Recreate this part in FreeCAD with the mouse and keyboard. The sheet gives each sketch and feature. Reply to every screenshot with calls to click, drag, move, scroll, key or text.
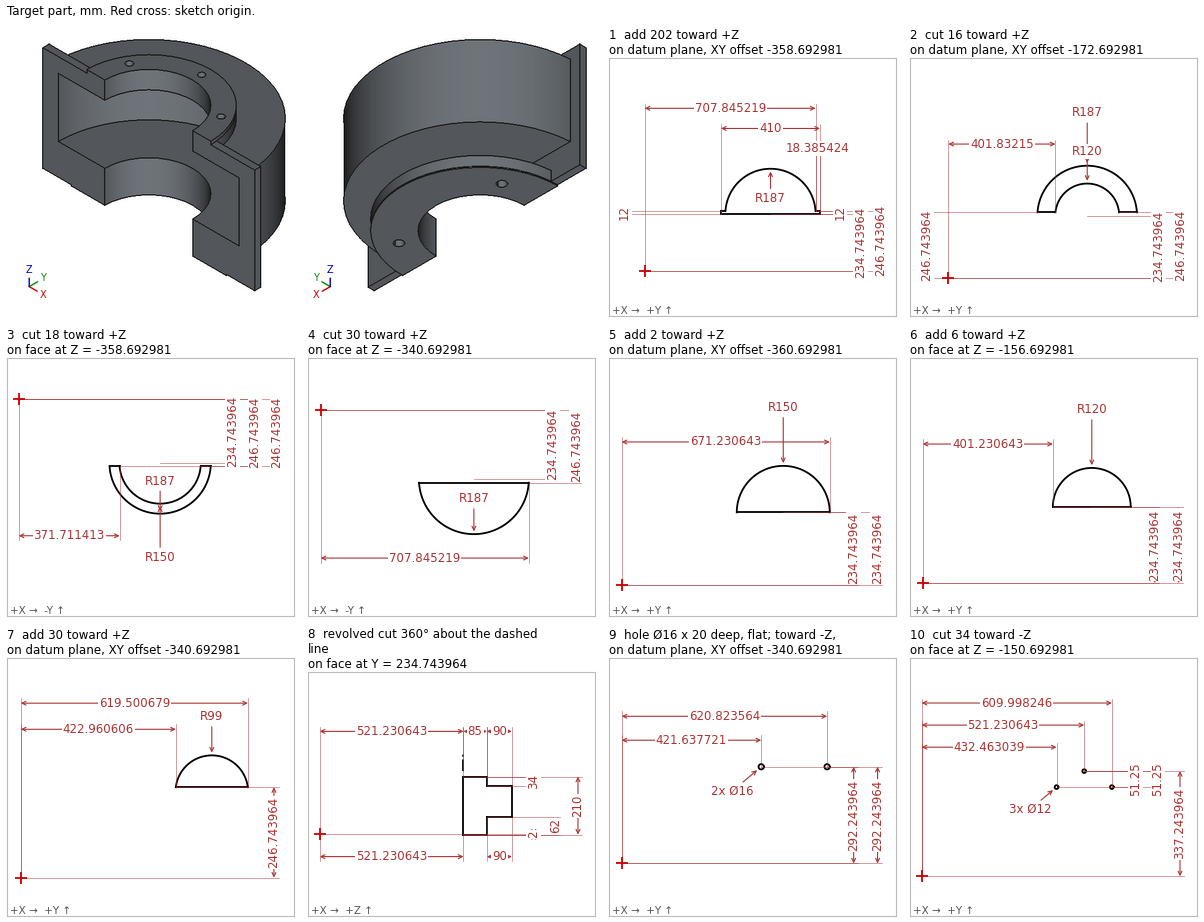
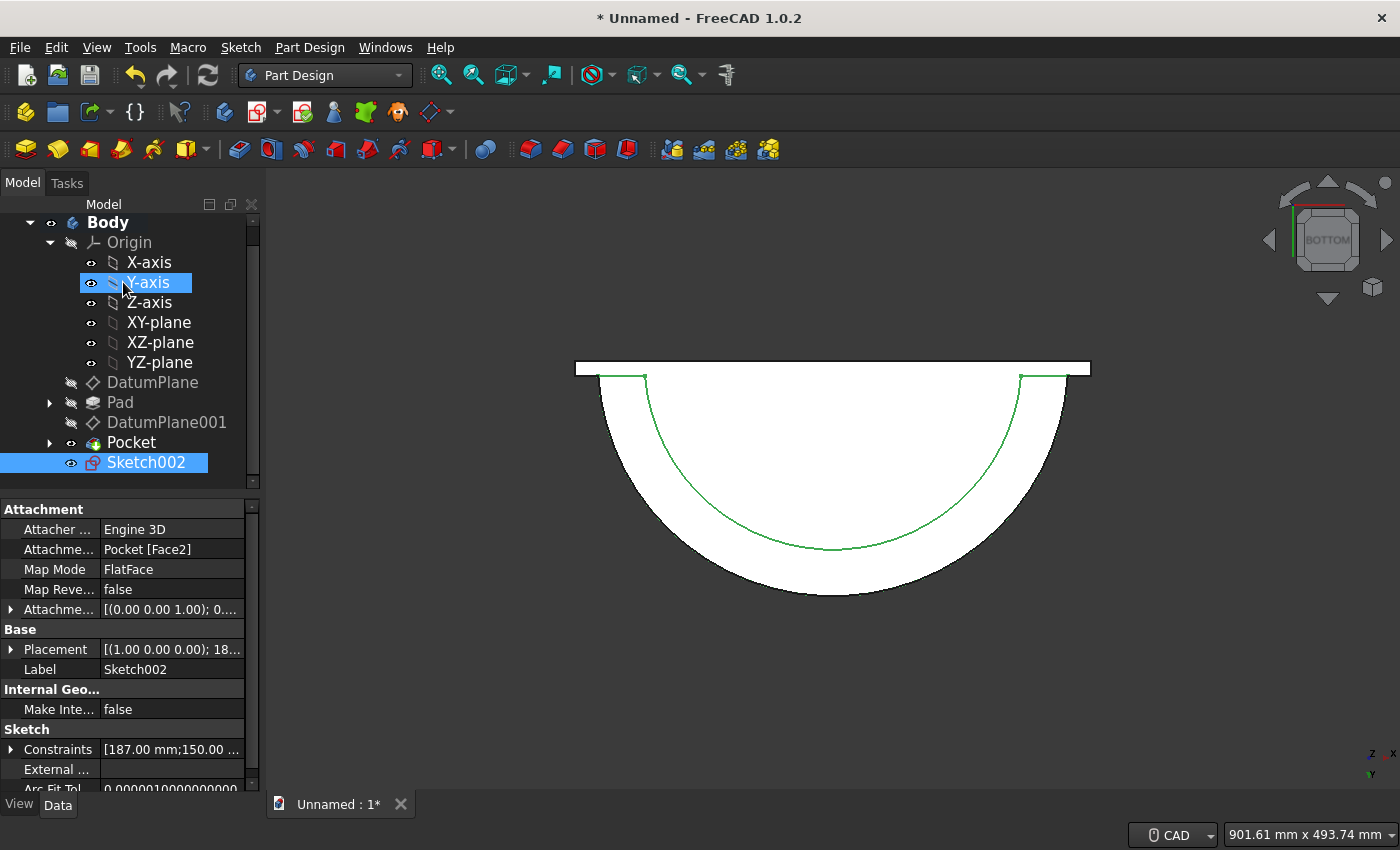
click(240, 150)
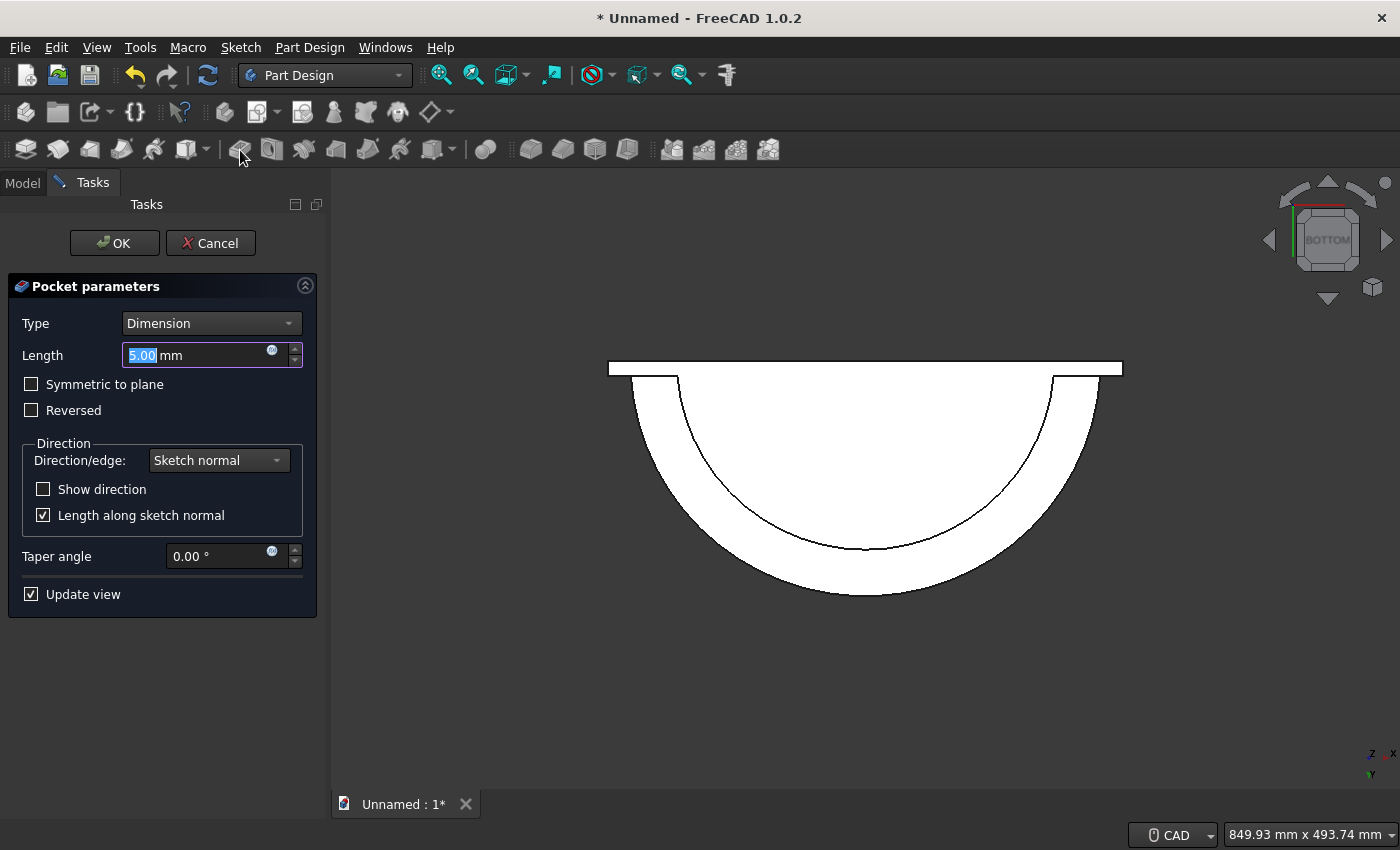
text(18)
key(Tab)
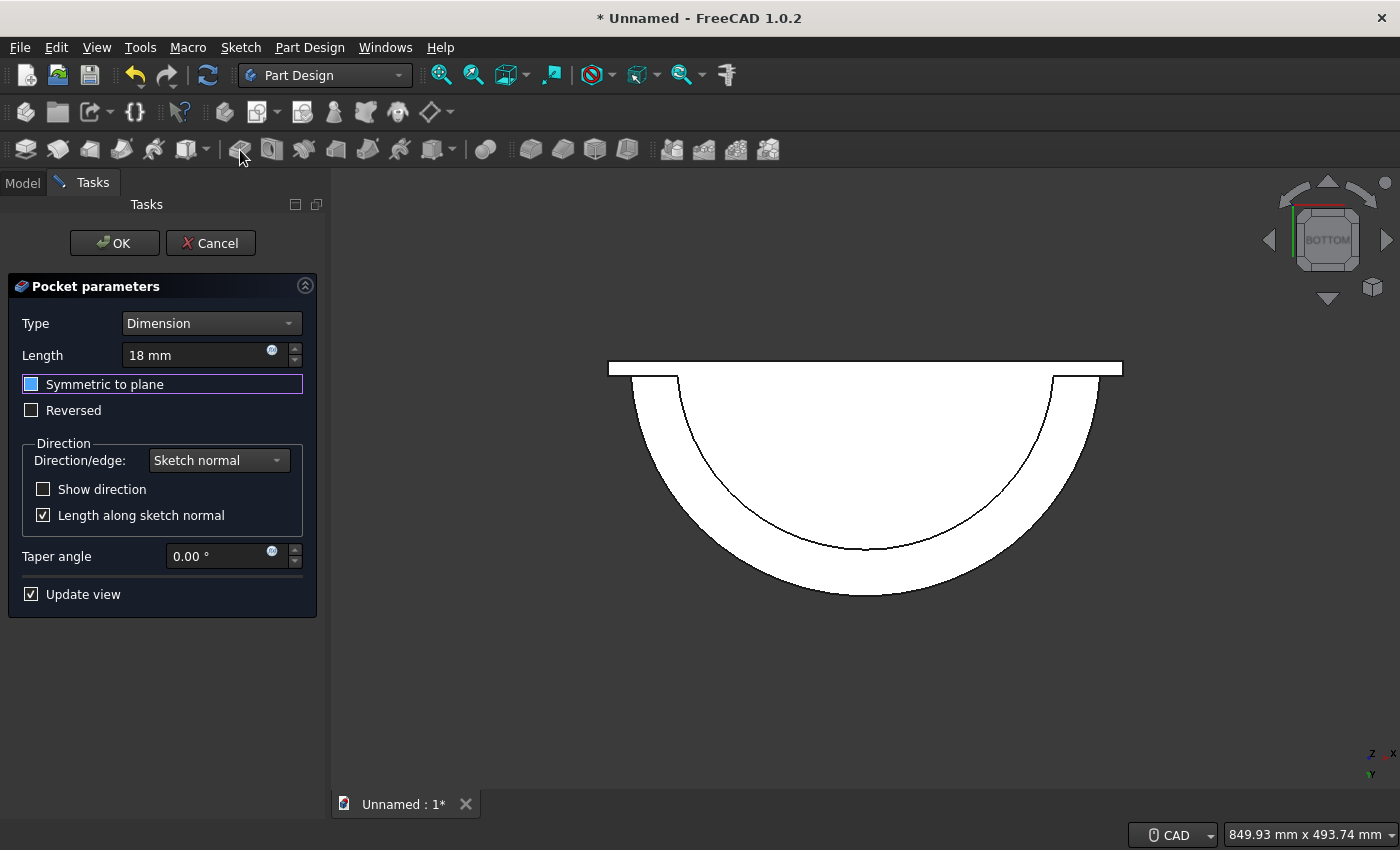
click(115, 243)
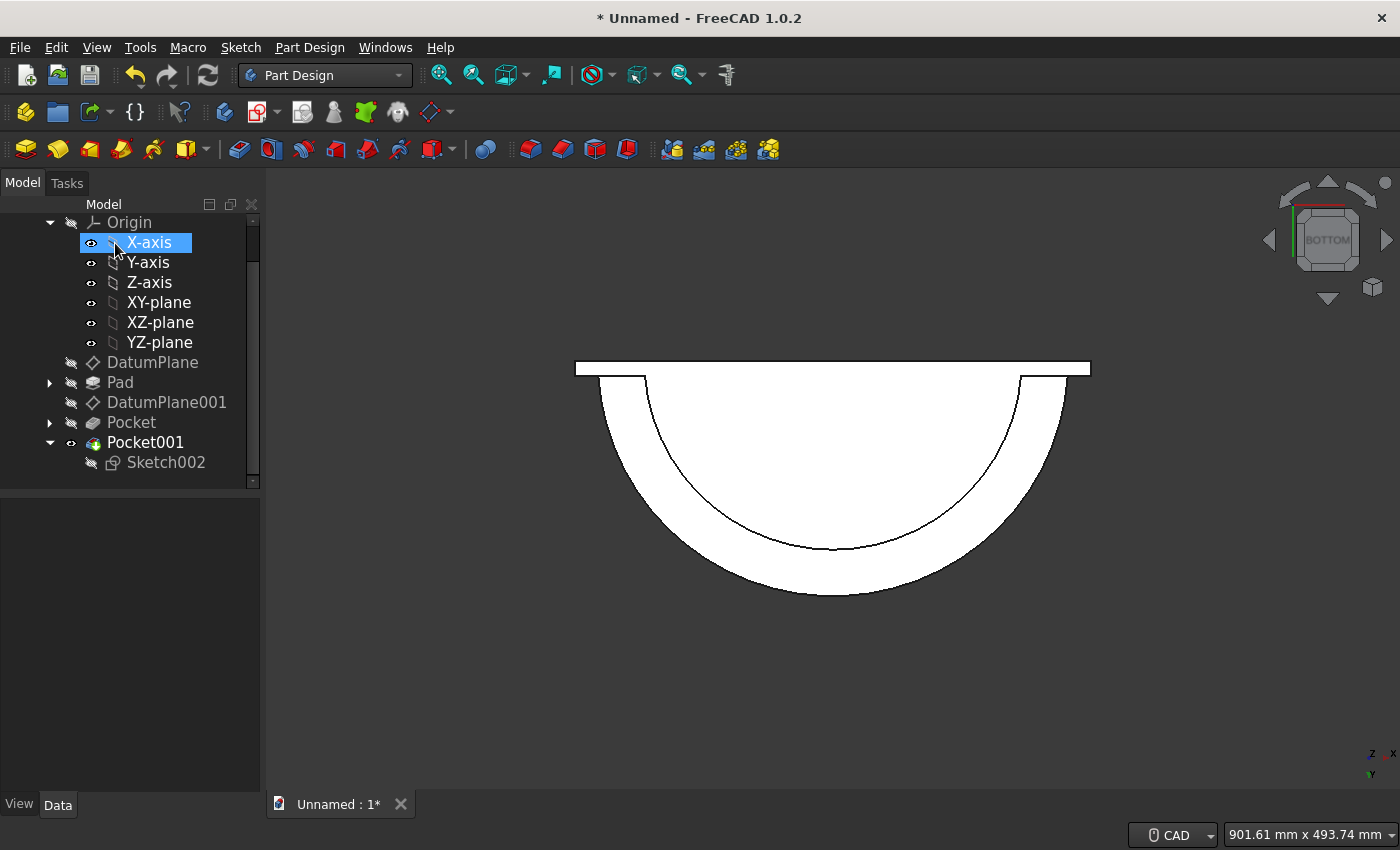
click(632, 422)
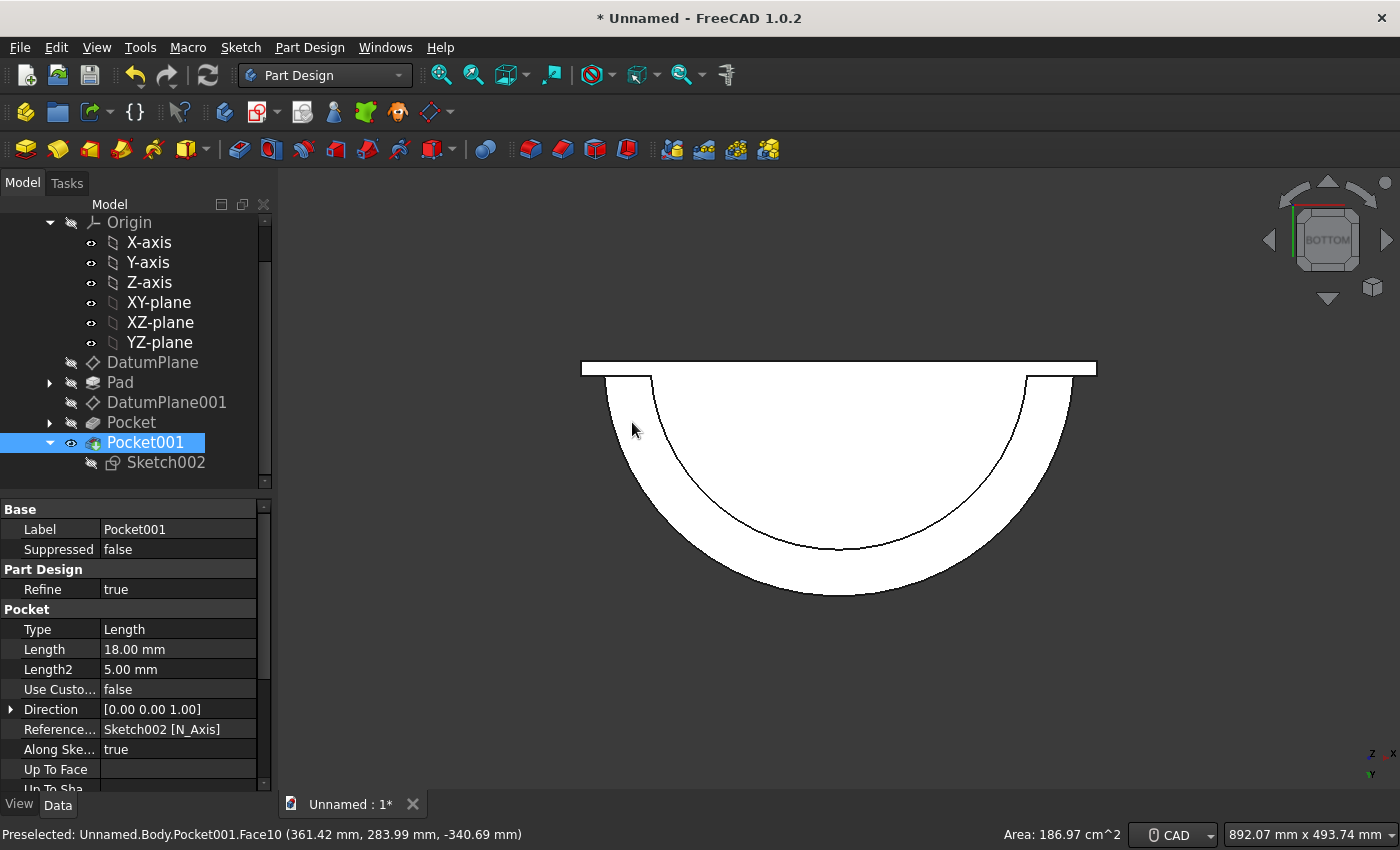
click(258, 112)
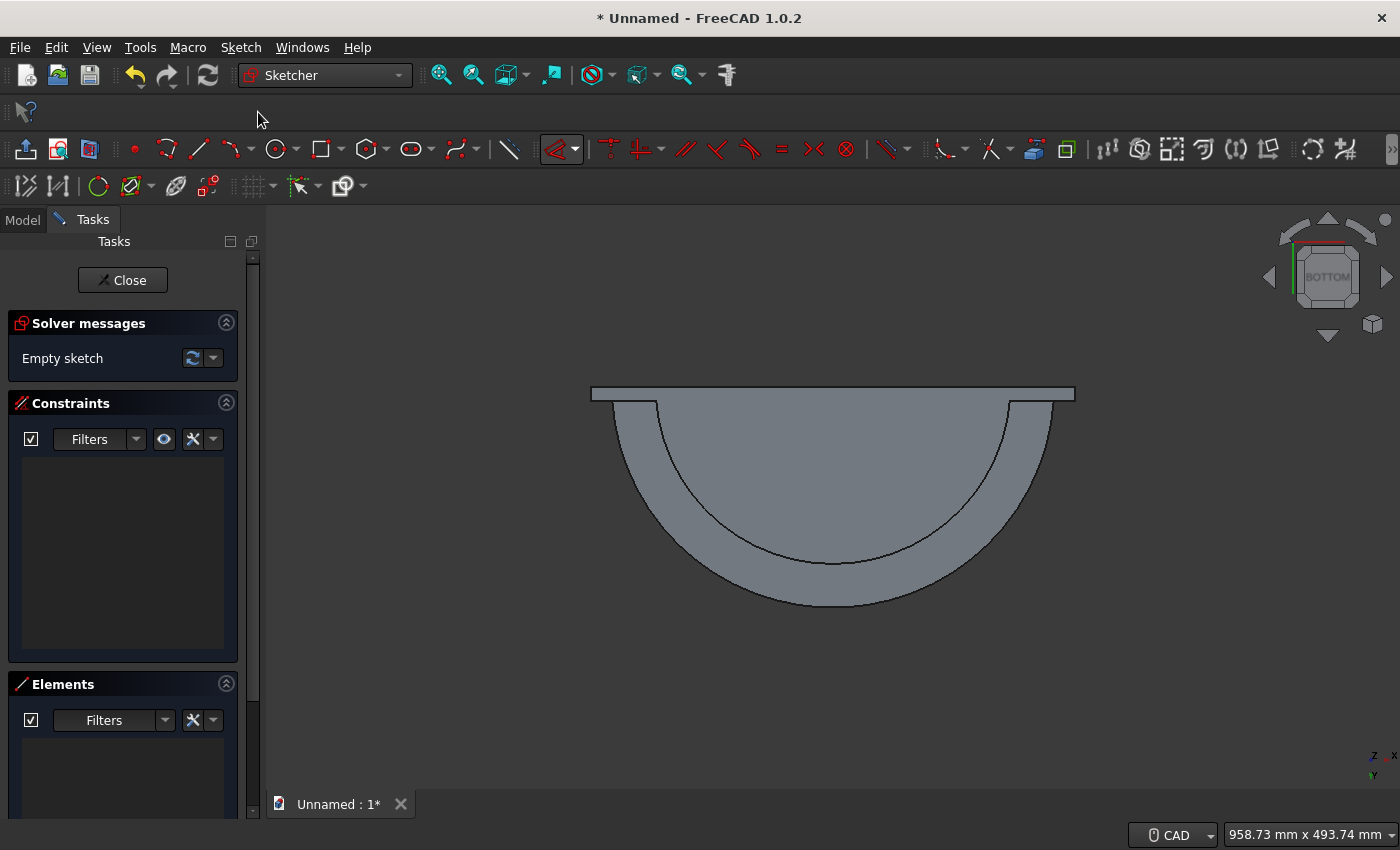
scroll(1028, 761, down, 2)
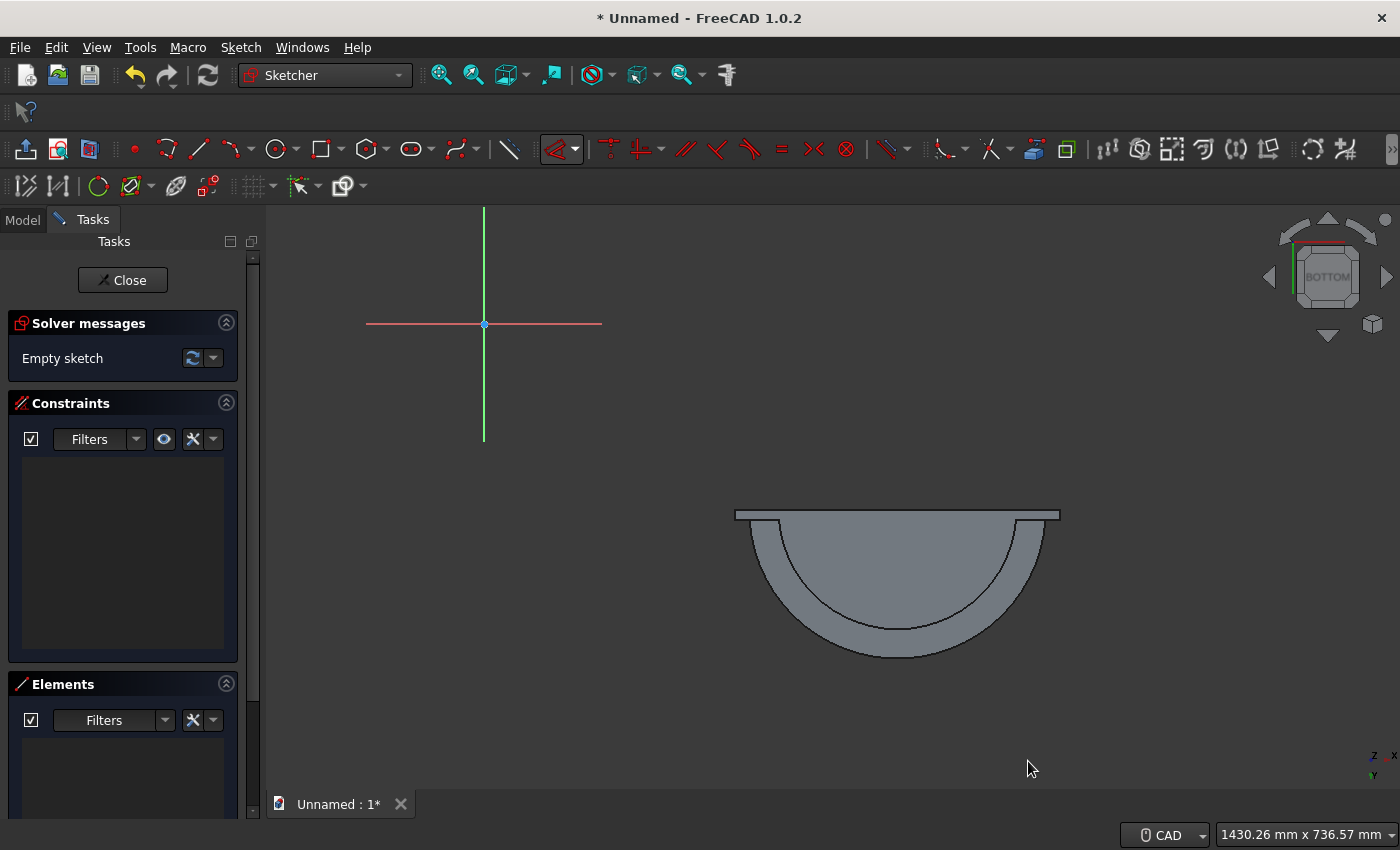
key(g)
key(l)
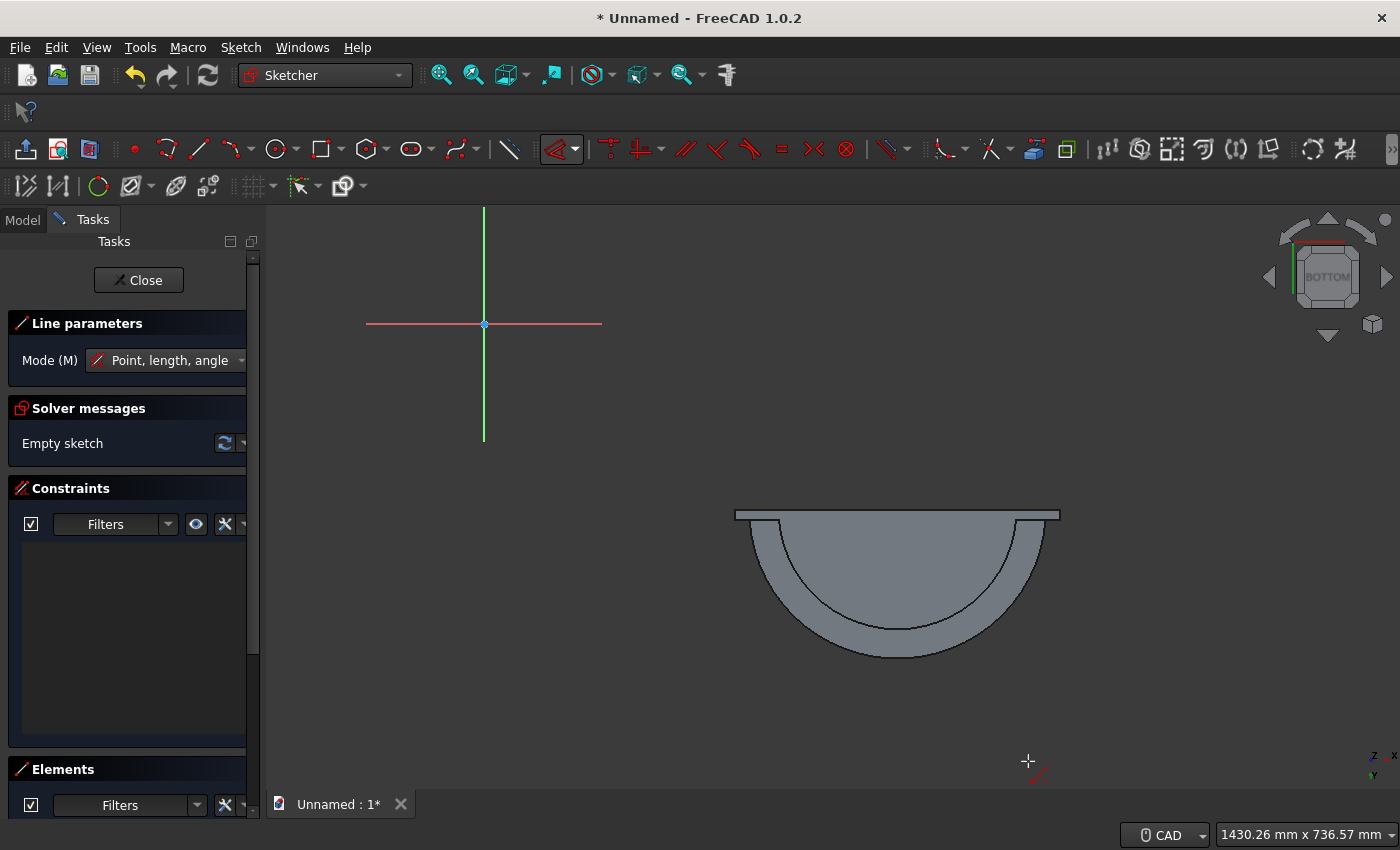
click(1045, 520)
click(750, 520)